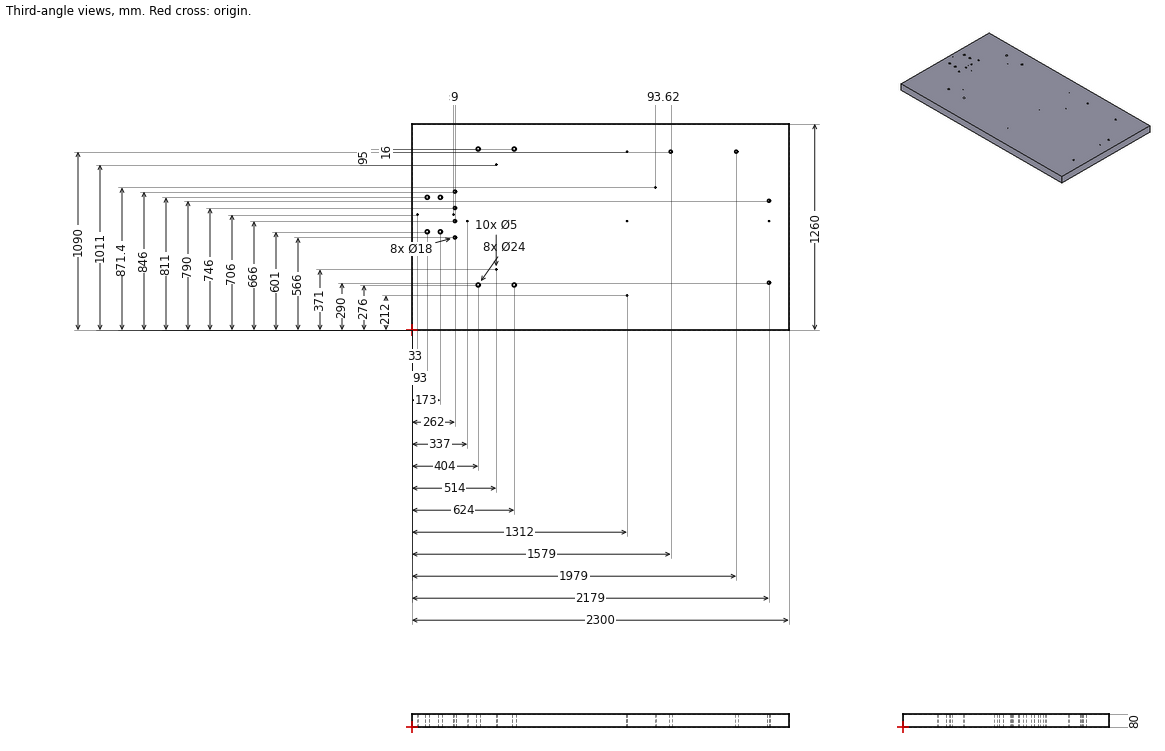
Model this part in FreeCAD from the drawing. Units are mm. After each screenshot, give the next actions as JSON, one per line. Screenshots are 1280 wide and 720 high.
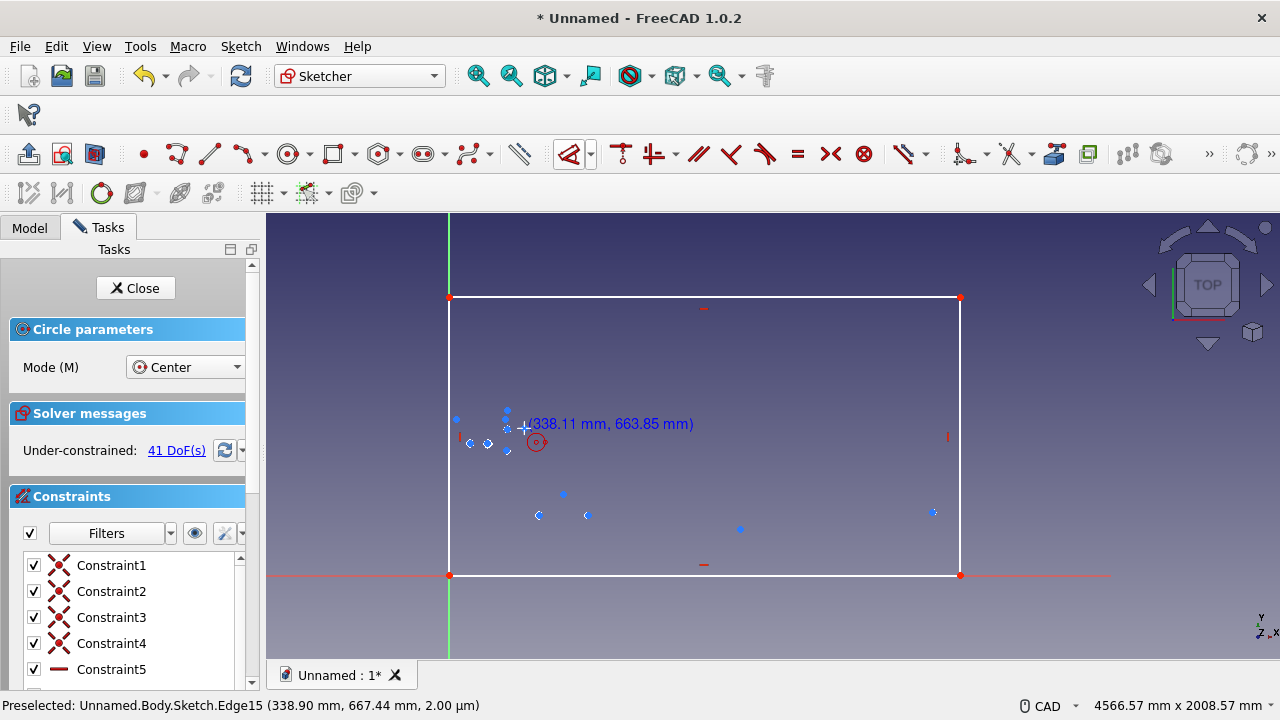
{"action": "scroll", "coordinate": [470, 396], "scroll_direction": "up", "scroll_amount": 11}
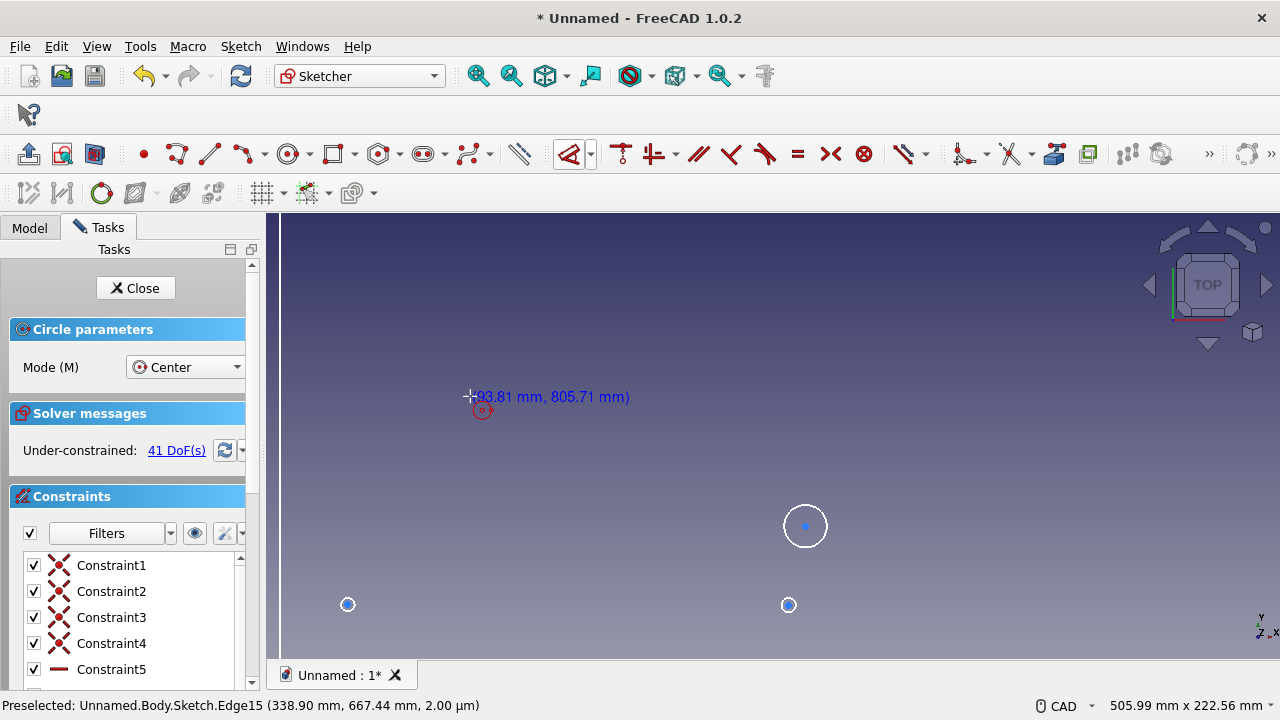
{"action": "scroll", "coordinate": [470, 396], "scroll_direction": "down", "scroll_amount": 11}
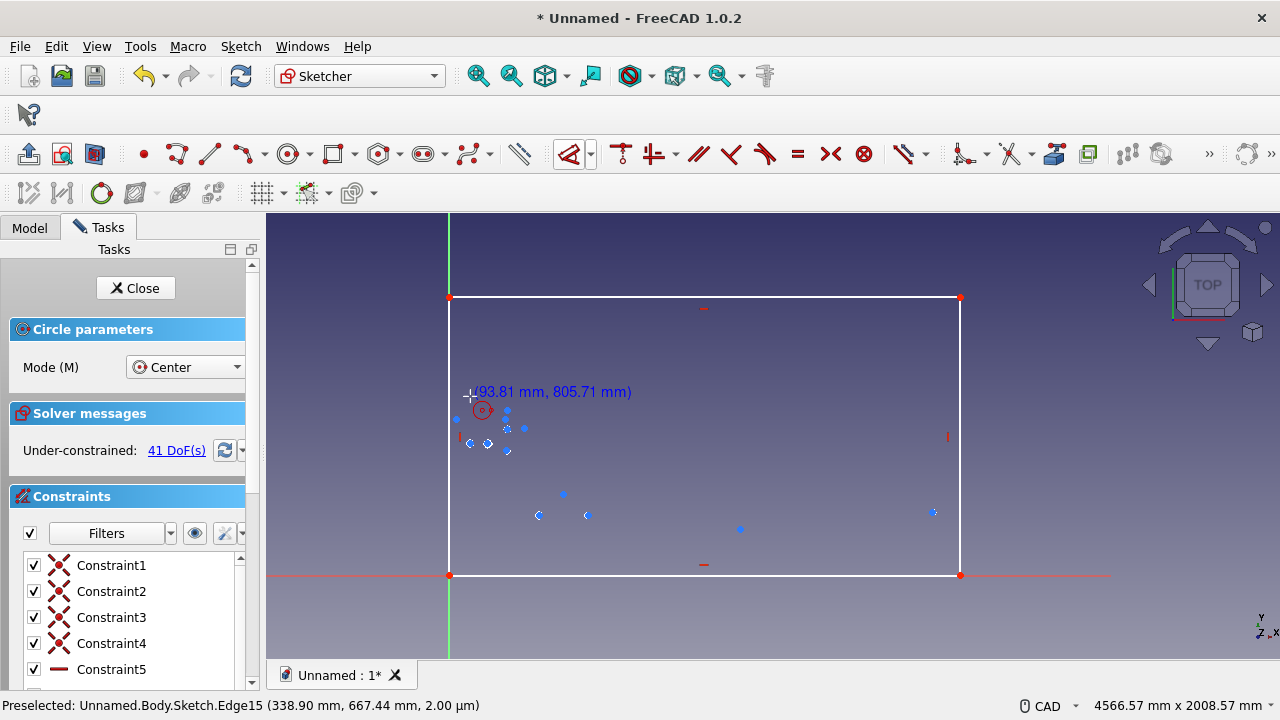
{"action": "left_click", "coordinate": [470, 396]}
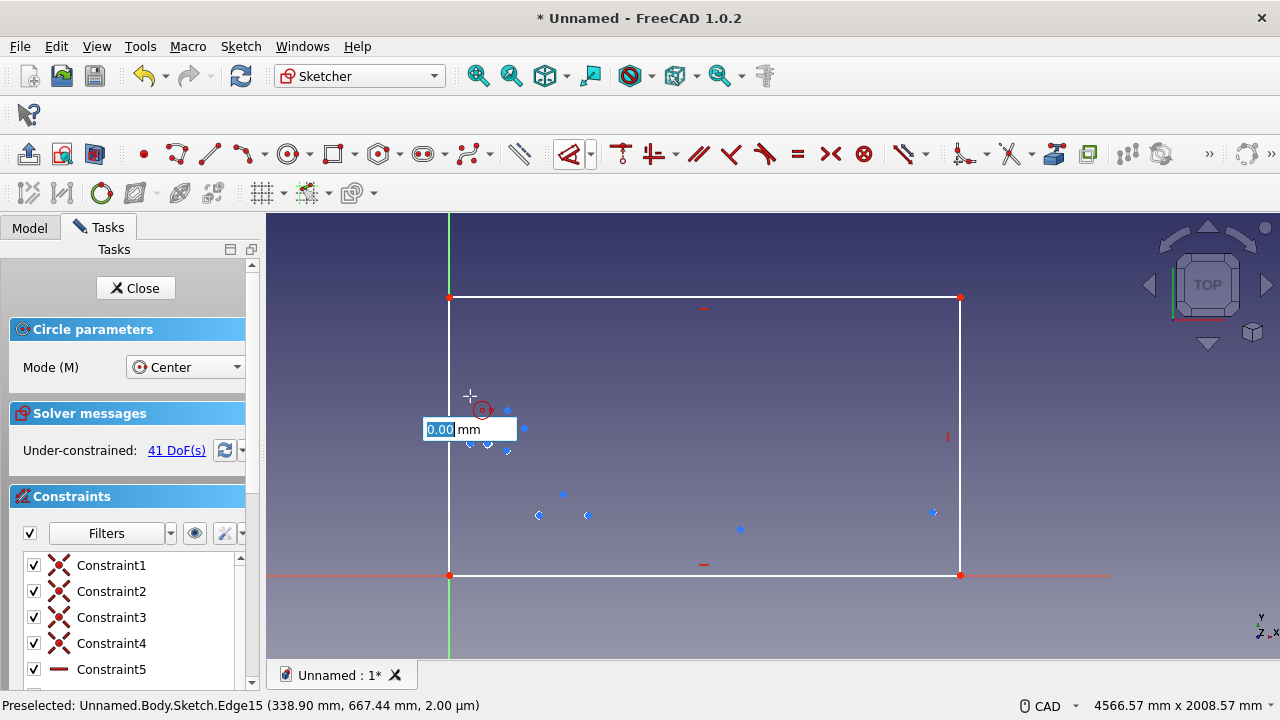
{"action": "scroll", "coordinate": [472, 394], "scroll_direction": "up", "scroll_amount": 9}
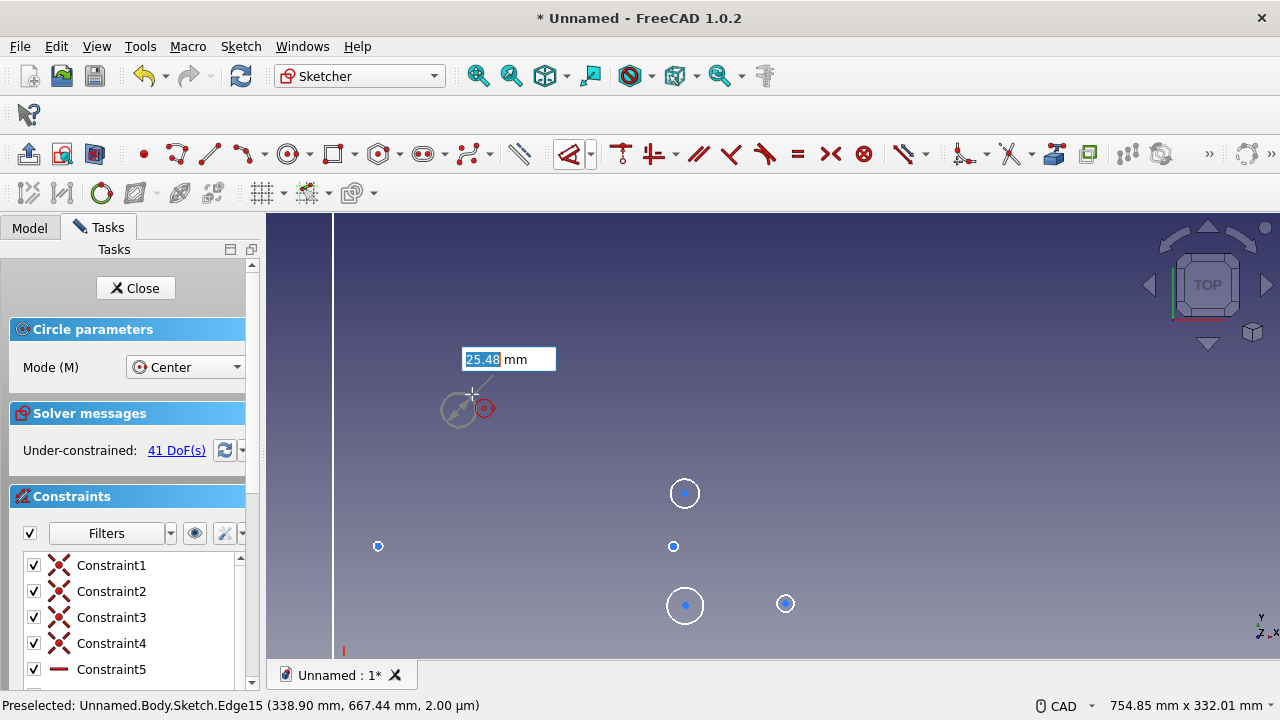
{"action": "left_click", "coordinate": [469, 392]}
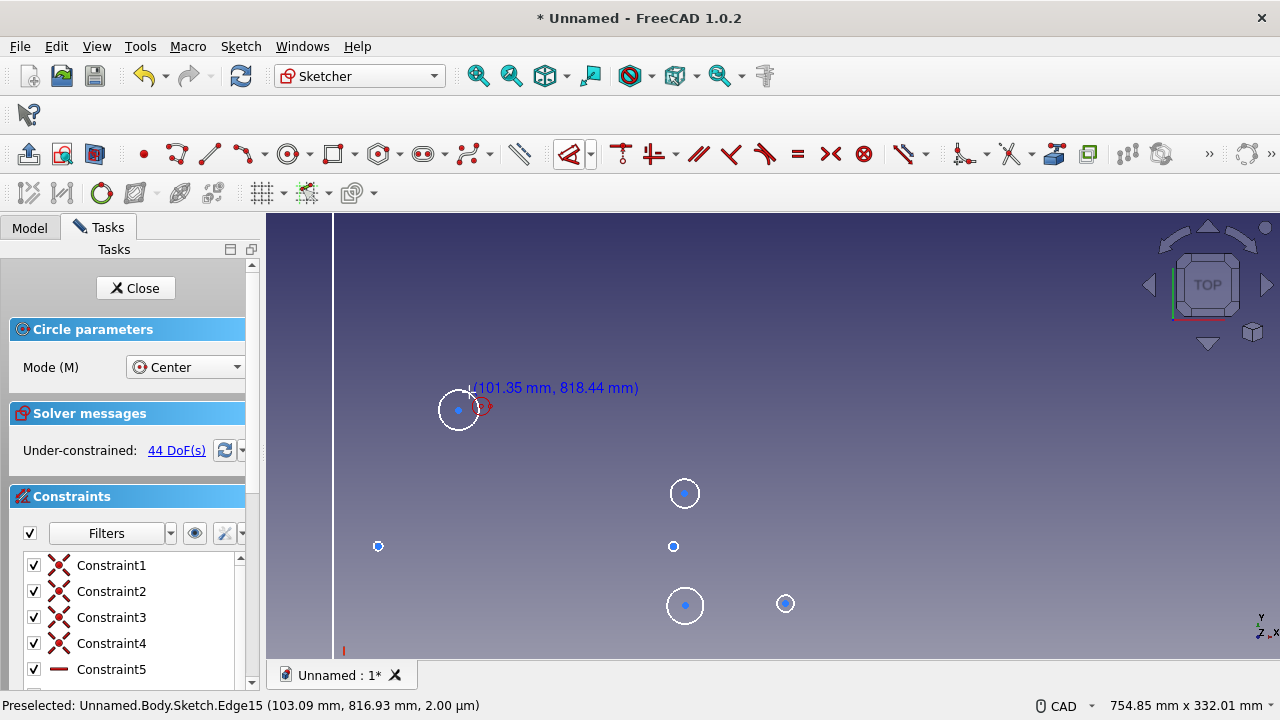
{"action": "scroll", "coordinate": [565, 403], "scroll_direction": "up", "scroll_amount": 2}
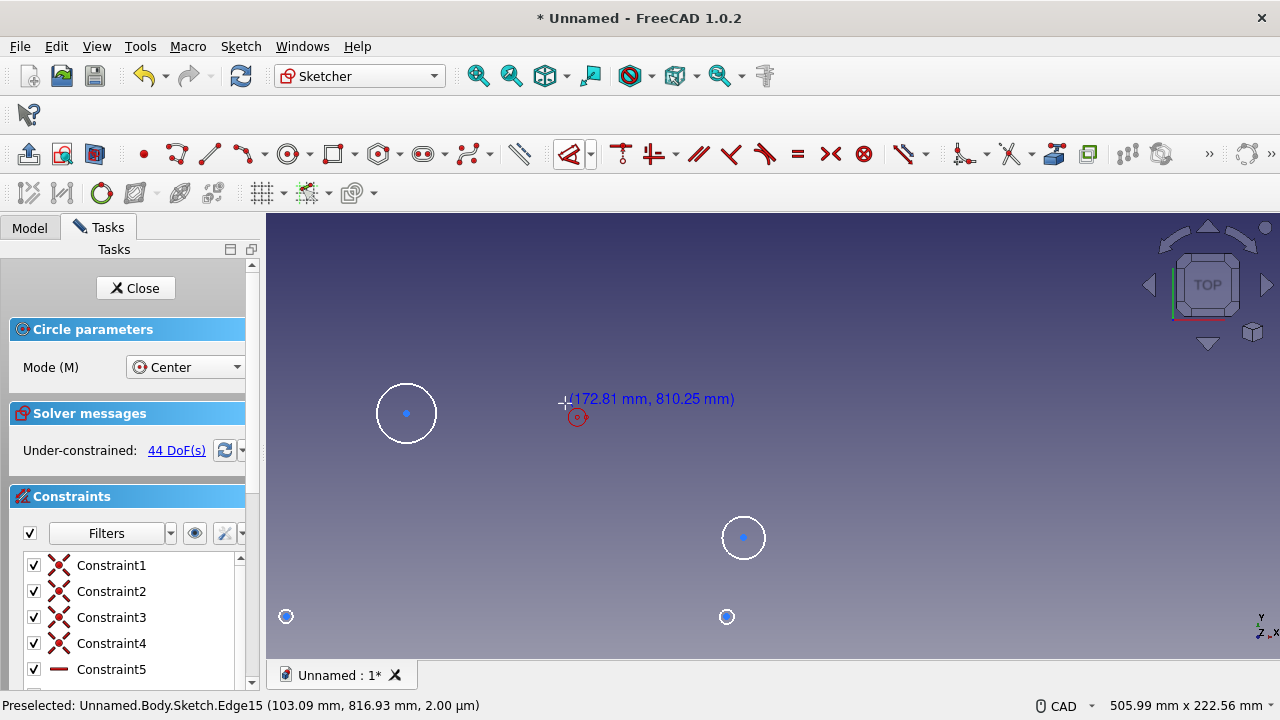
{"action": "scroll", "coordinate": [478, 395], "scroll_direction": "down", "scroll_amount": 11}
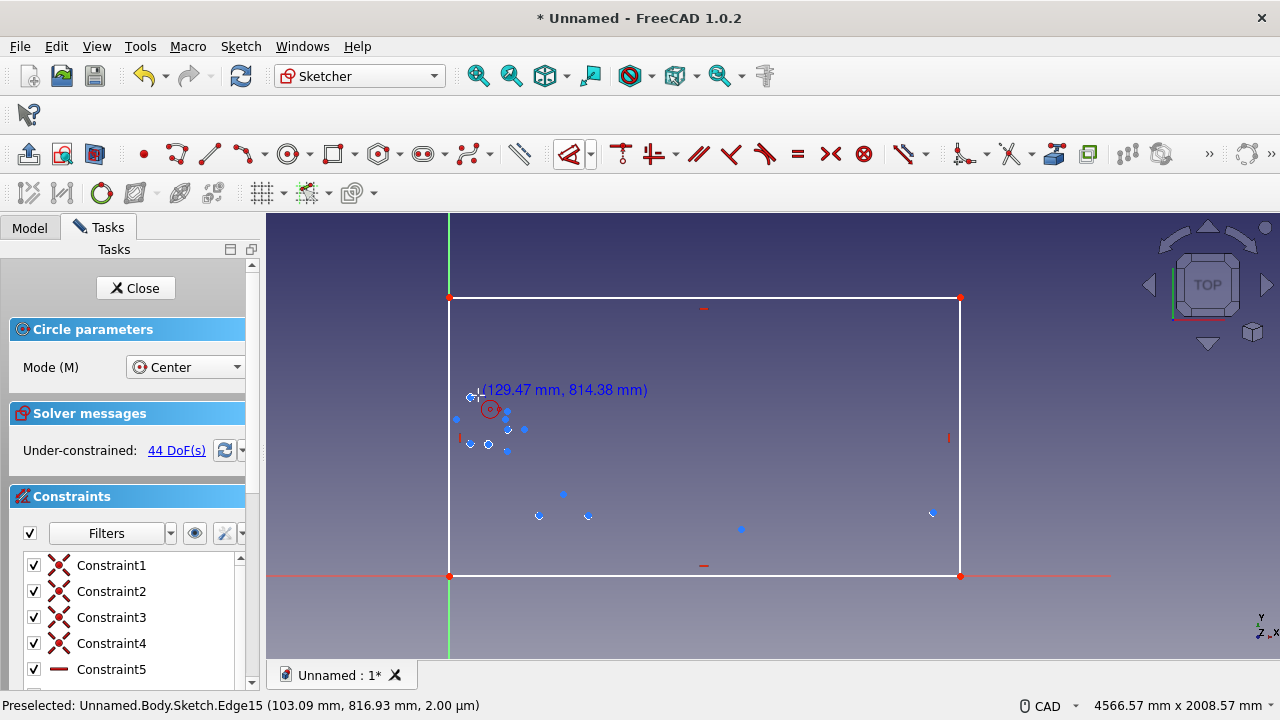
{"action": "left_click", "coordinate": [488, 396]}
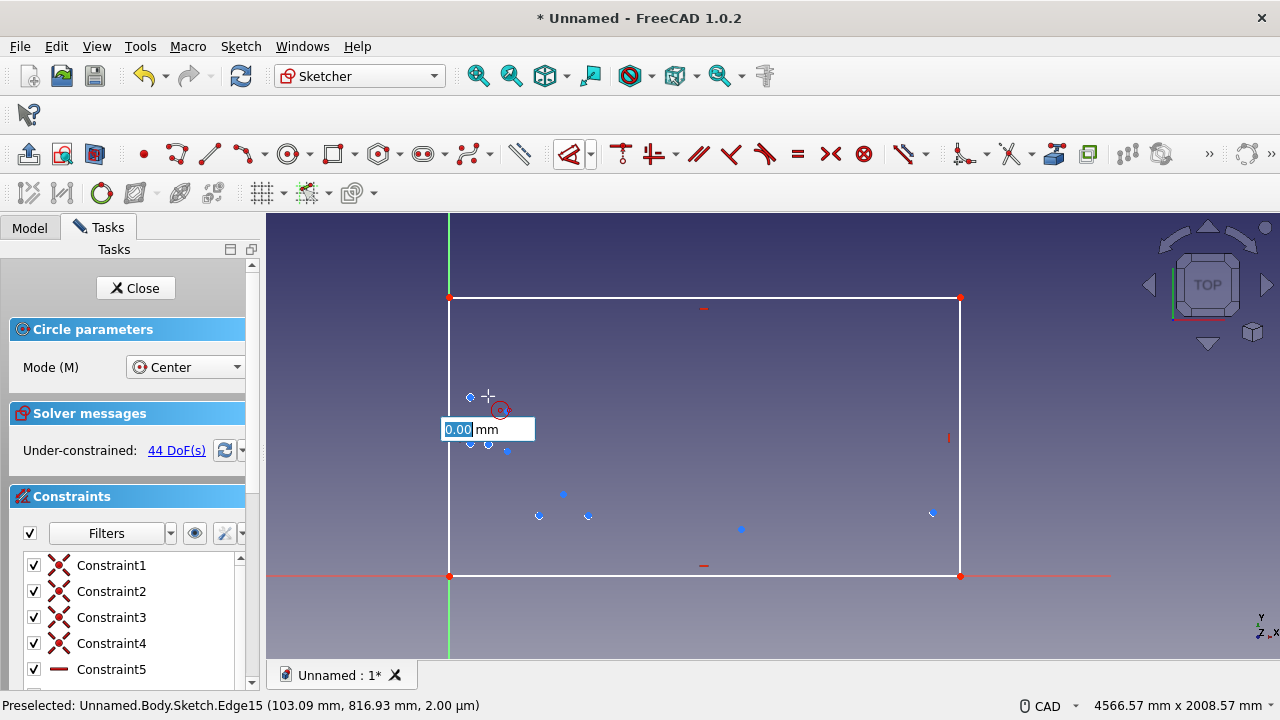
{"action": "scroll", "coordinate": [490, 394], "scroll_direction": "up", "scroll_amount": 9}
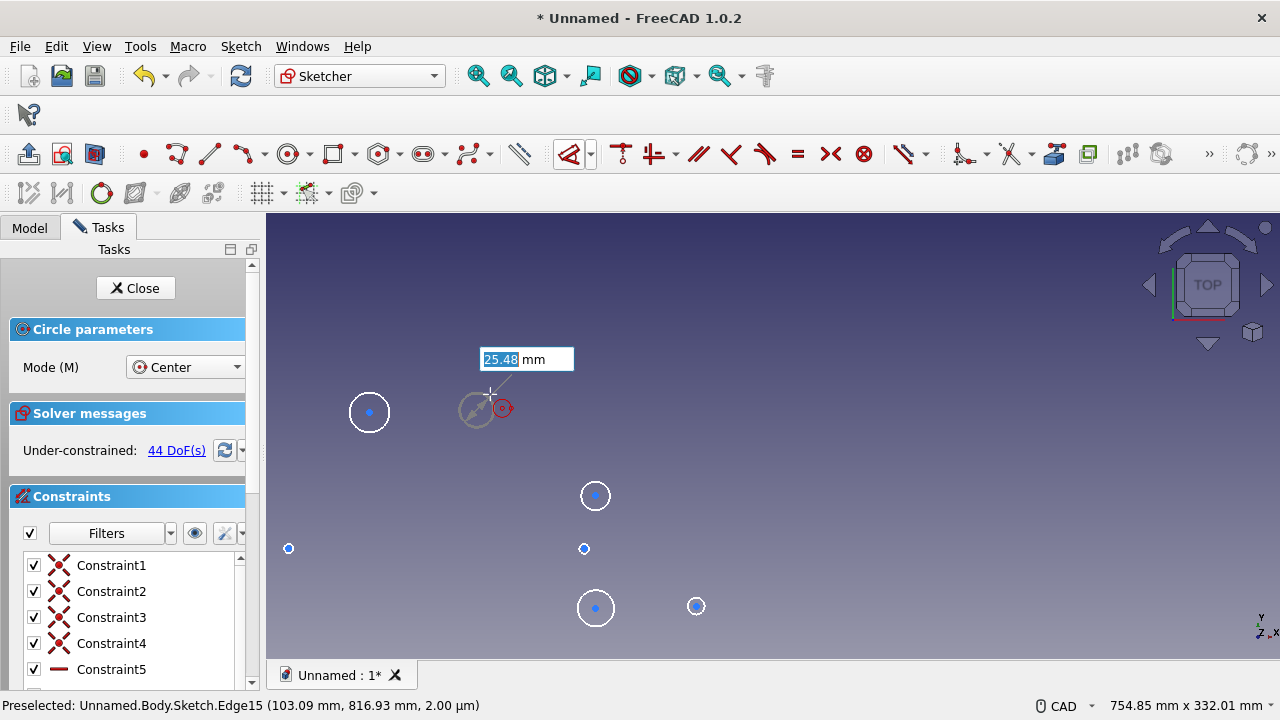
{"action": "left_click", "coordinate": [487, 394]}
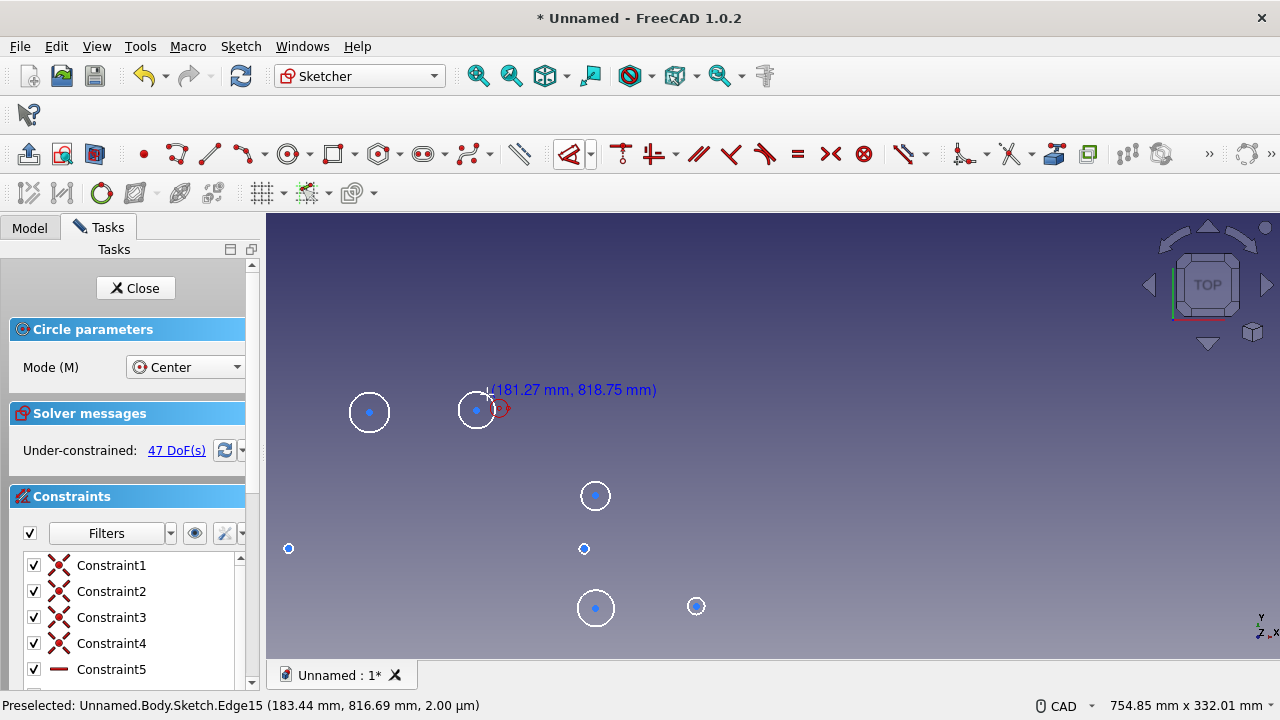
{"action": "scroll", "coordinate": [595, 358], "scroll_direction": "up", "scroll_amount": 4}